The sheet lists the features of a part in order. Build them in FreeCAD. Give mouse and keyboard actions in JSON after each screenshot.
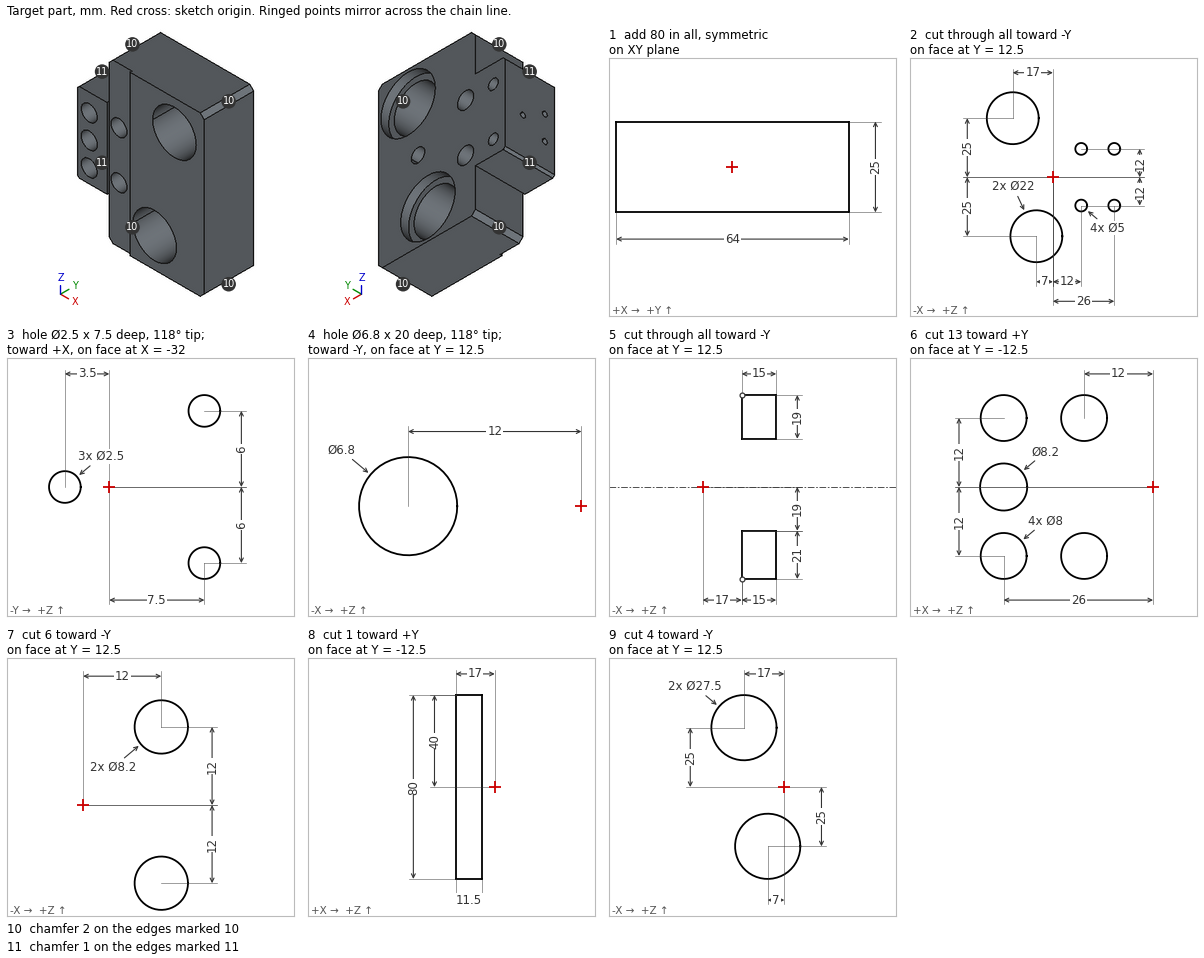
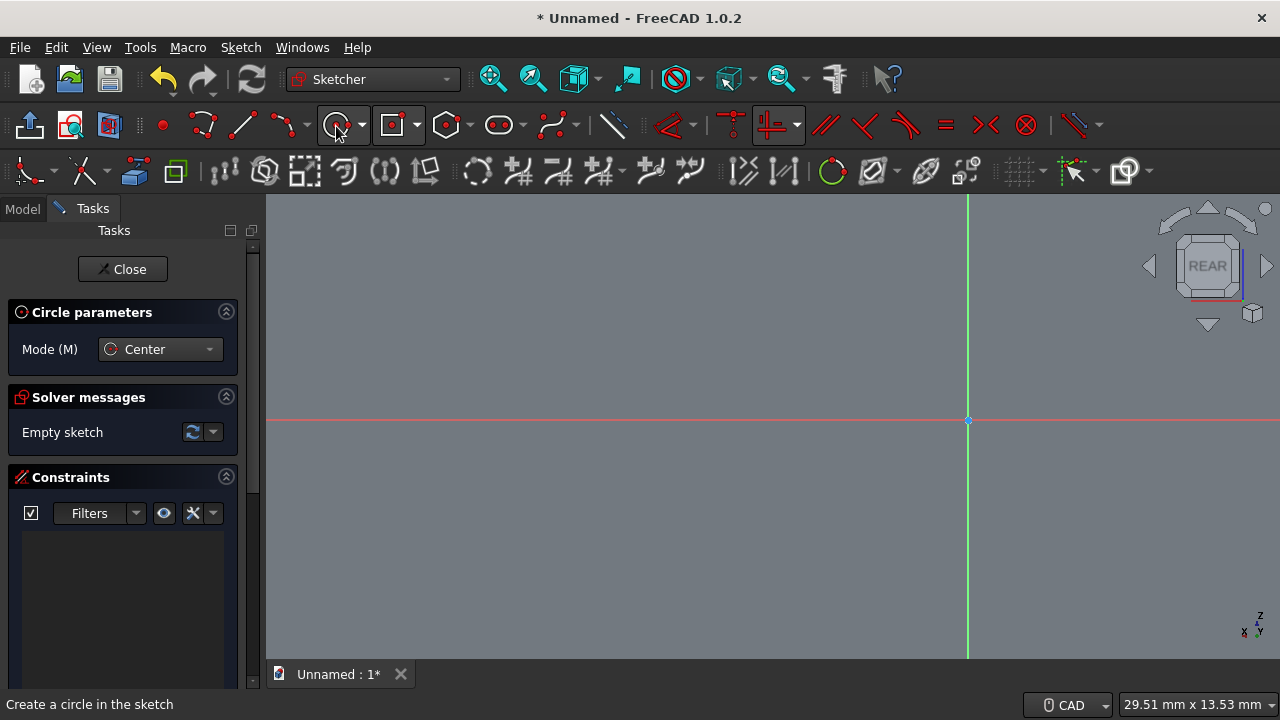
{"action": "left_click", "coordinate": [556, 420]}
{"action": "left_click", "coordinate": [638, 337]}
{"action": "key", "text": "Escape"}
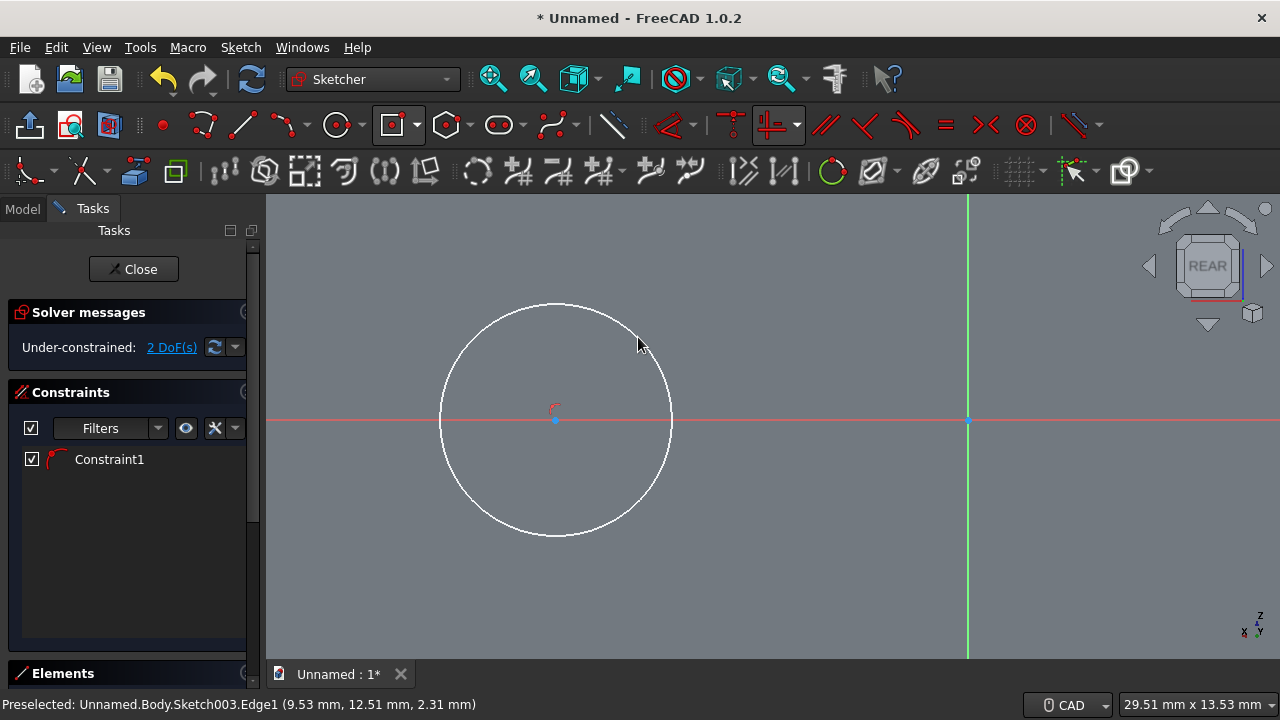
{"action": "left_click", "coordinate": [668, 126]}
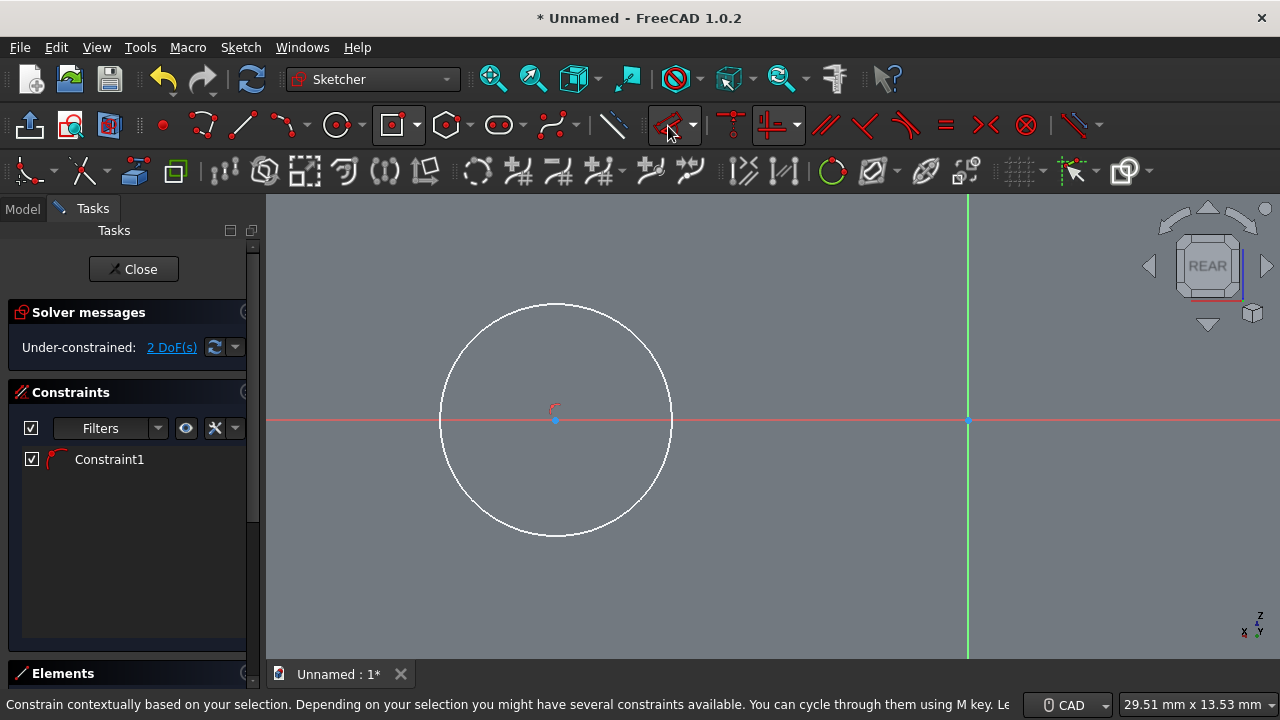
{"action": "left_click", "coordinate": [638, 338]}
{"action": "left_click", "coordinate": [661, 315]}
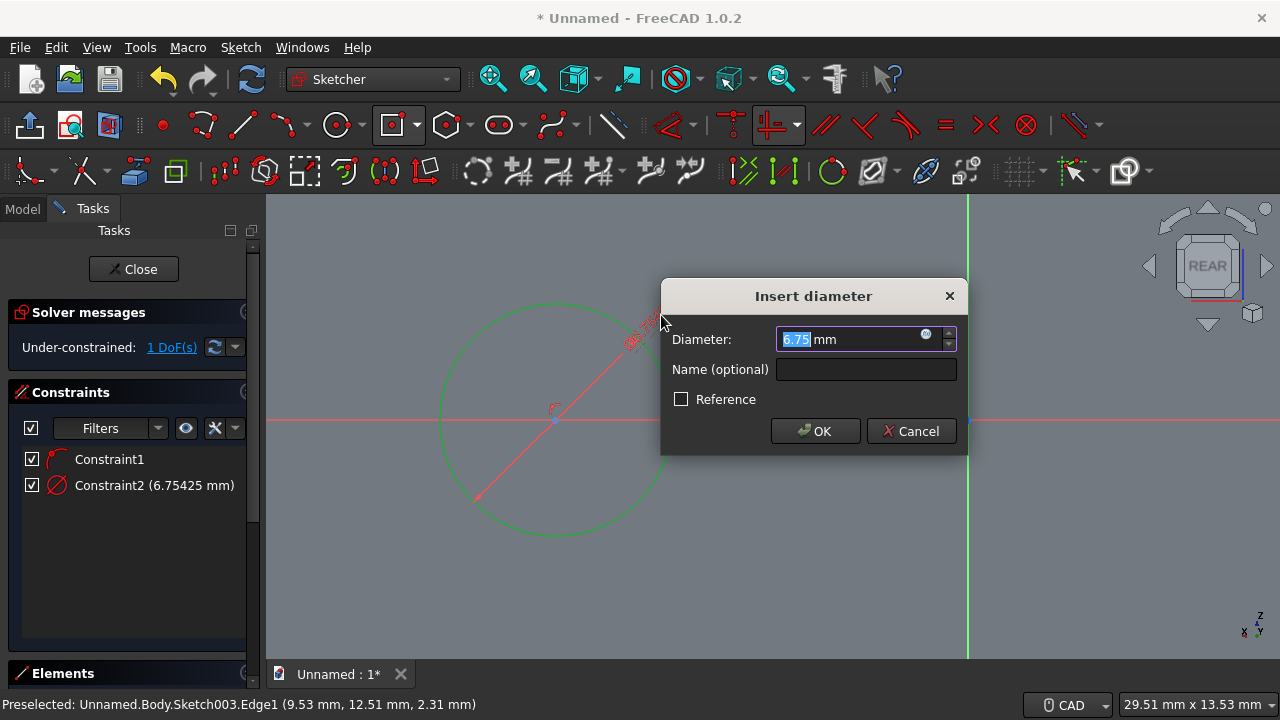
{"action": "type", "text": "6.8"}
{"action": "key", "text": "Return"}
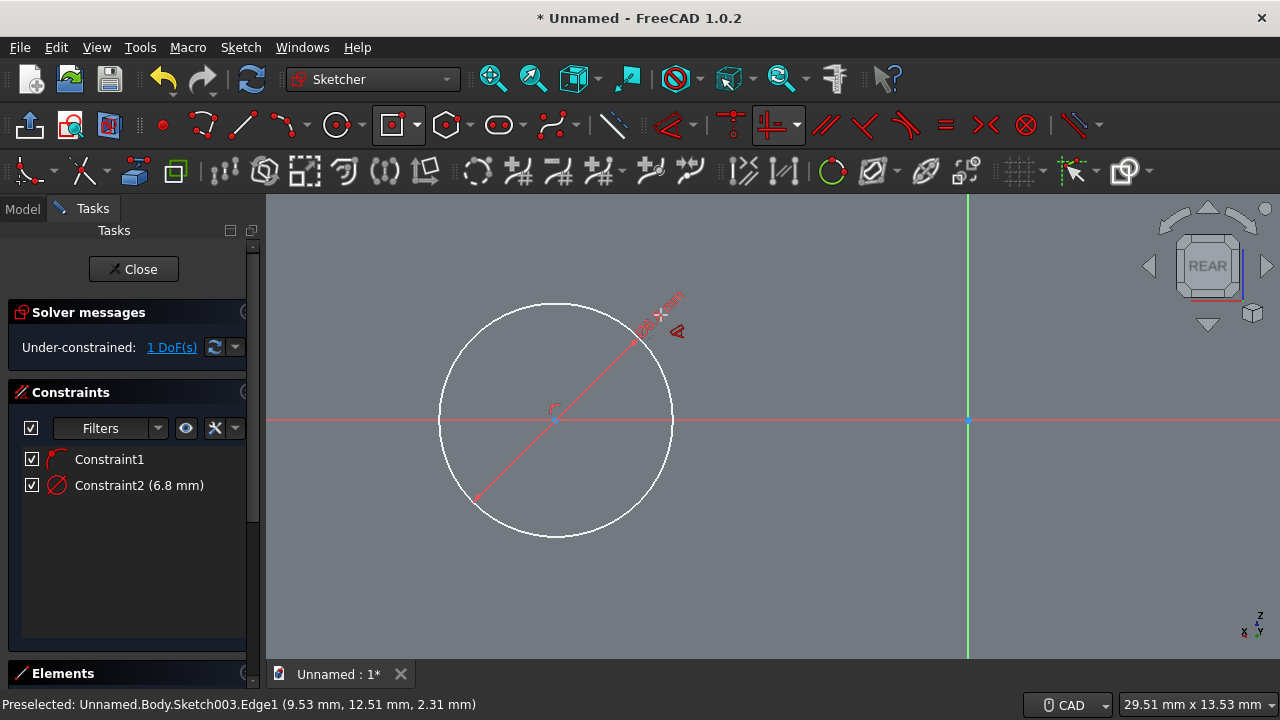
{"action": "left_click", "coordinate": [556, 420]}
{"action": "left_click", "coordinate": [762, 454]}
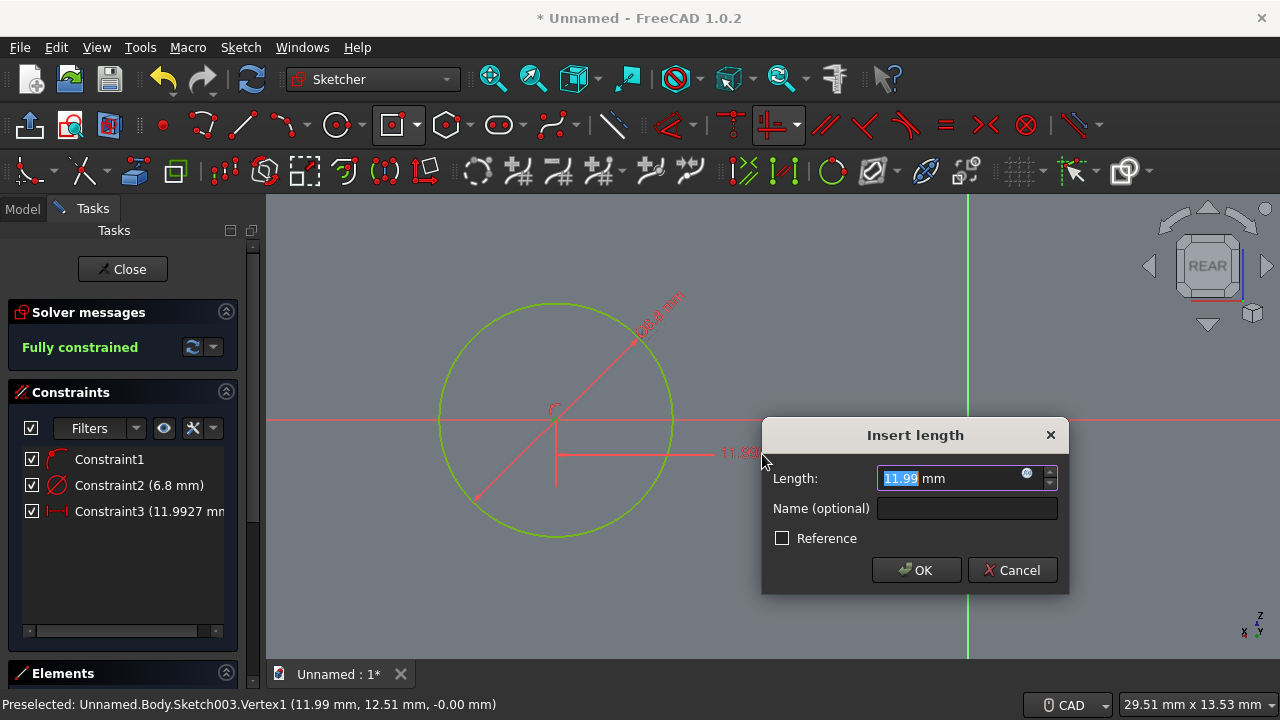
{"action": "type", "text": "12"}
{"action": "key", "text": "Return"}
{"action": "key", "text": "Escape"}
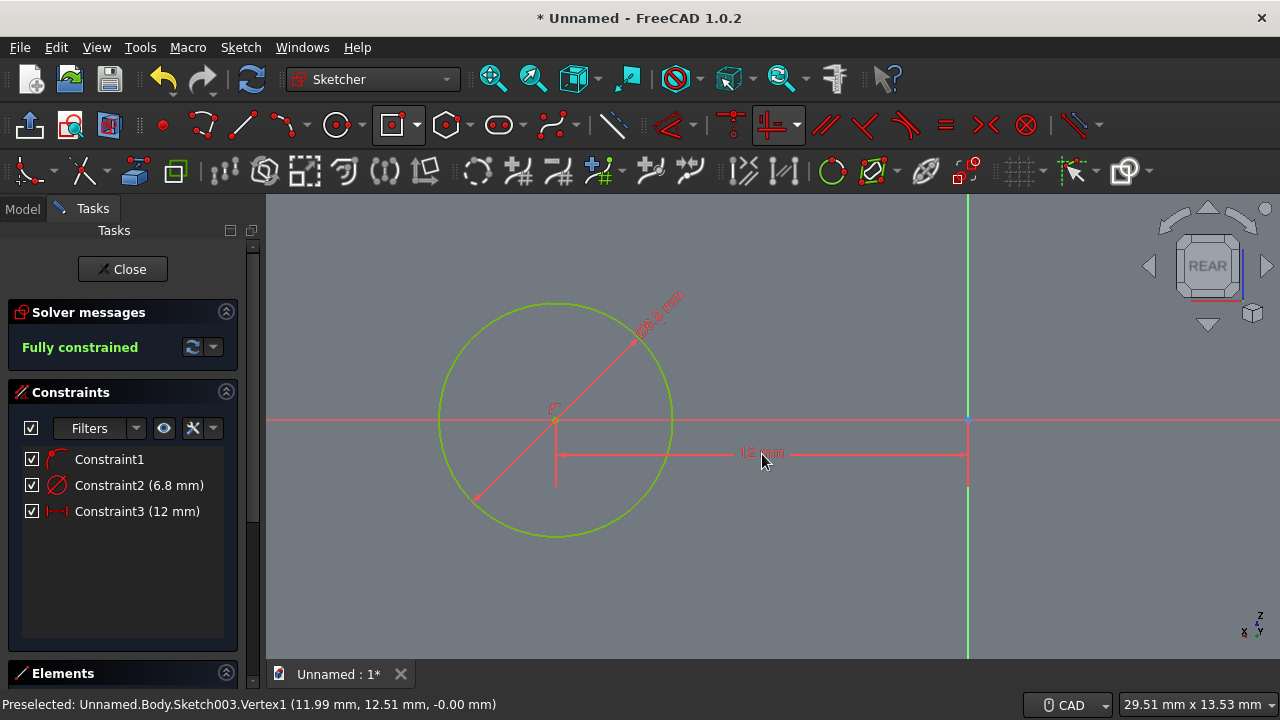
{"action": "left_click", "coordinate": [123, 269]}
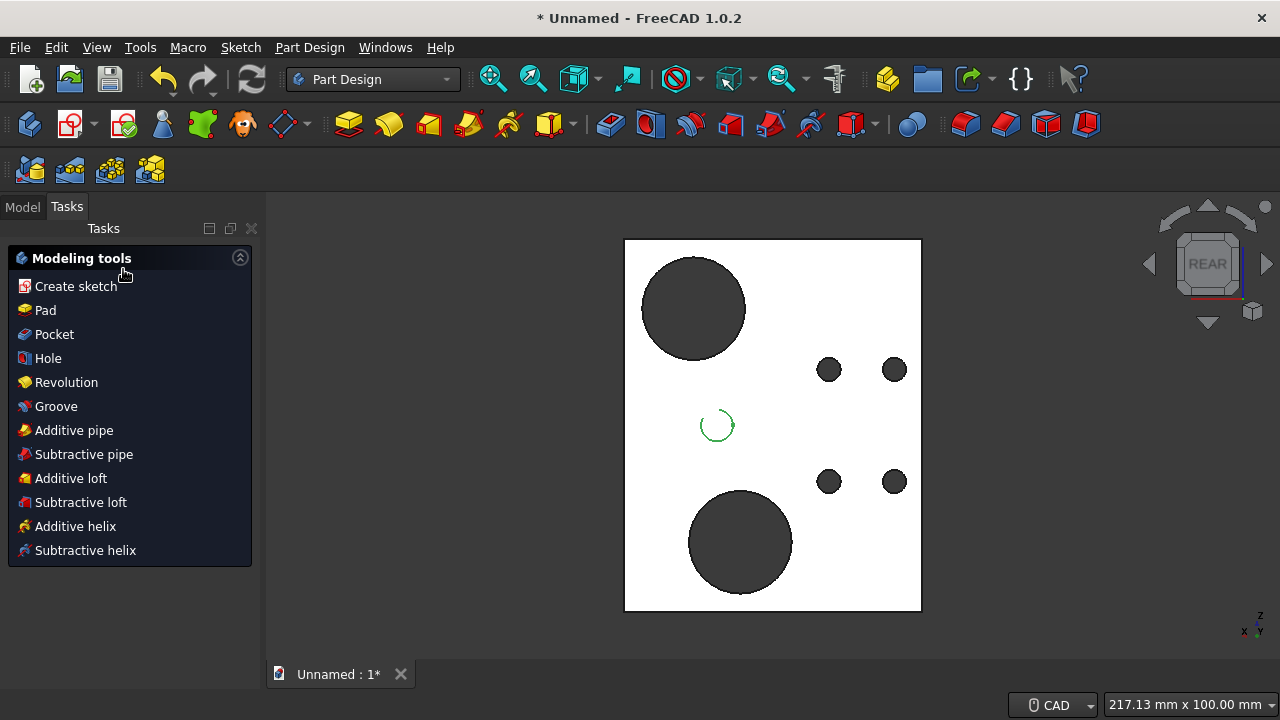
{"action": "left_click", "coordinate": [652, 124]}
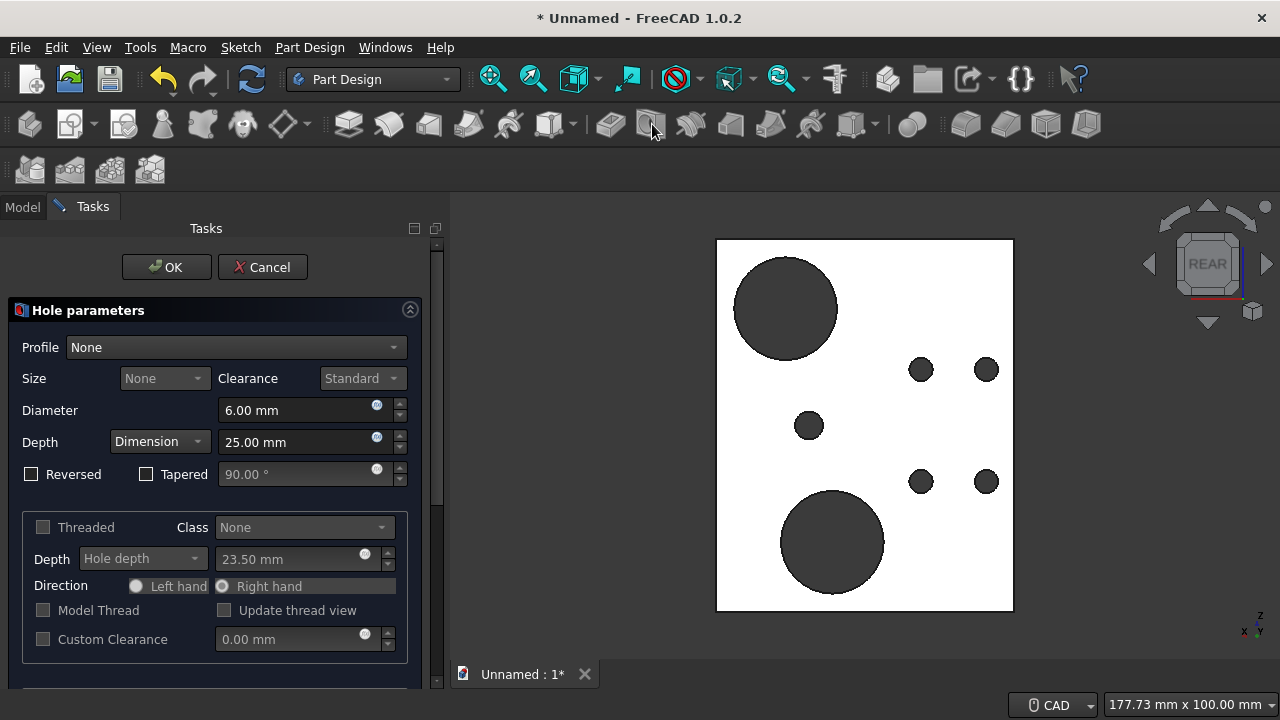
{"action": "triple_click", "coordinate": [305, 410]}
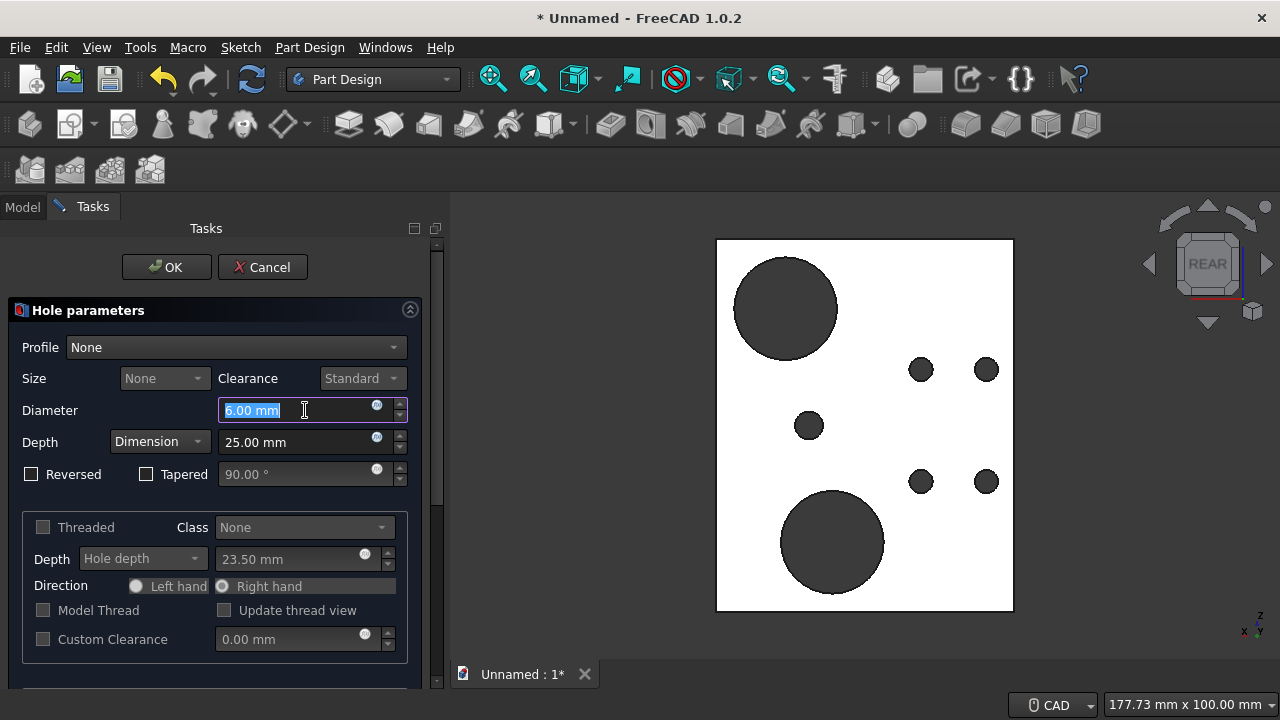
{"action": "type", "text": "6.8"}
{"action": "key", "text": "Tab"}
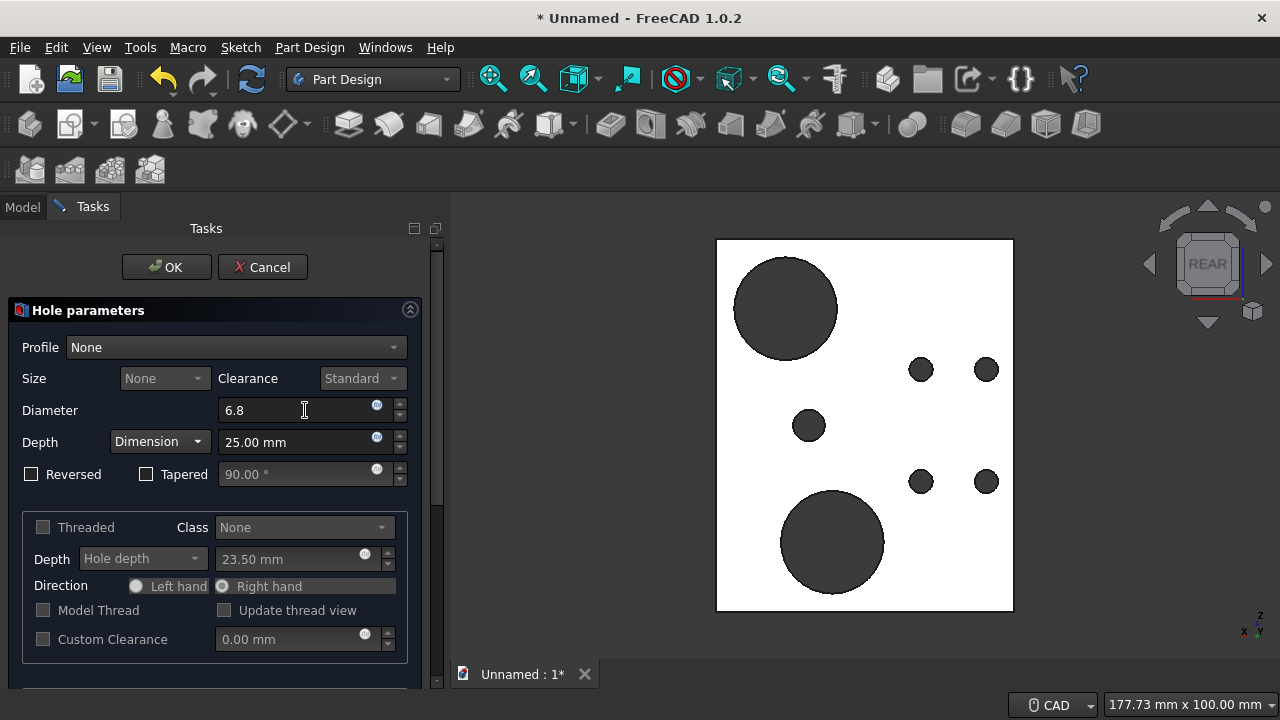
{"action": "triple_click", "coordinate": [305, 442]}